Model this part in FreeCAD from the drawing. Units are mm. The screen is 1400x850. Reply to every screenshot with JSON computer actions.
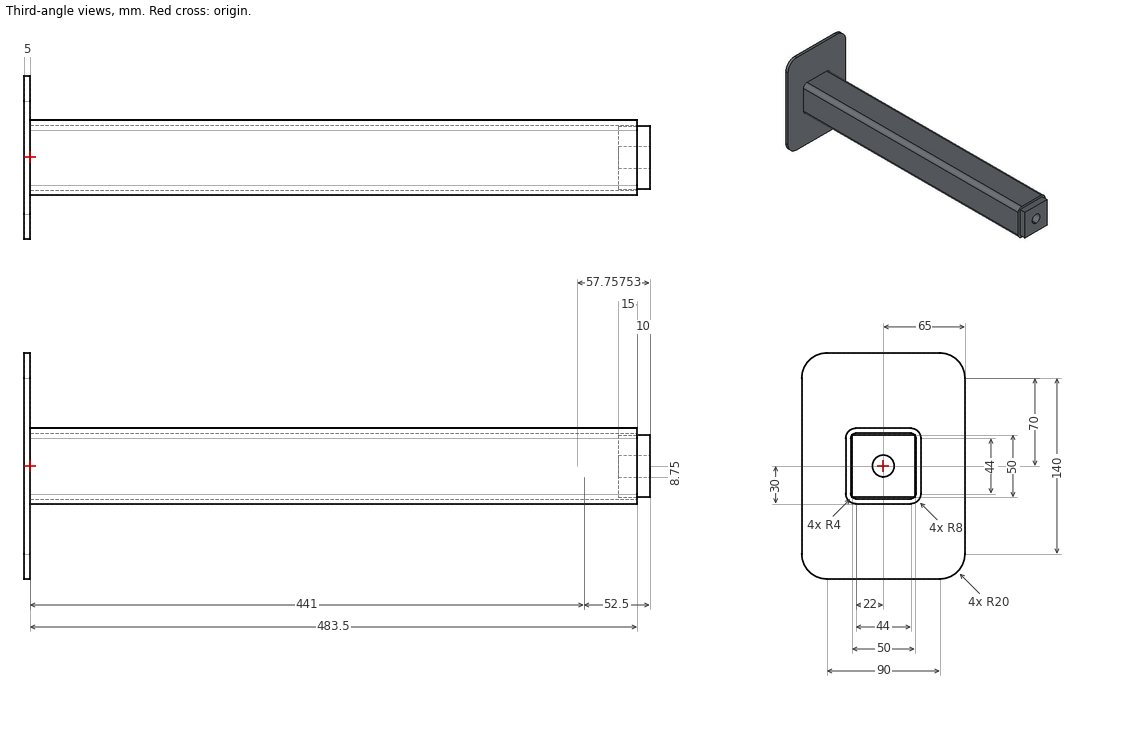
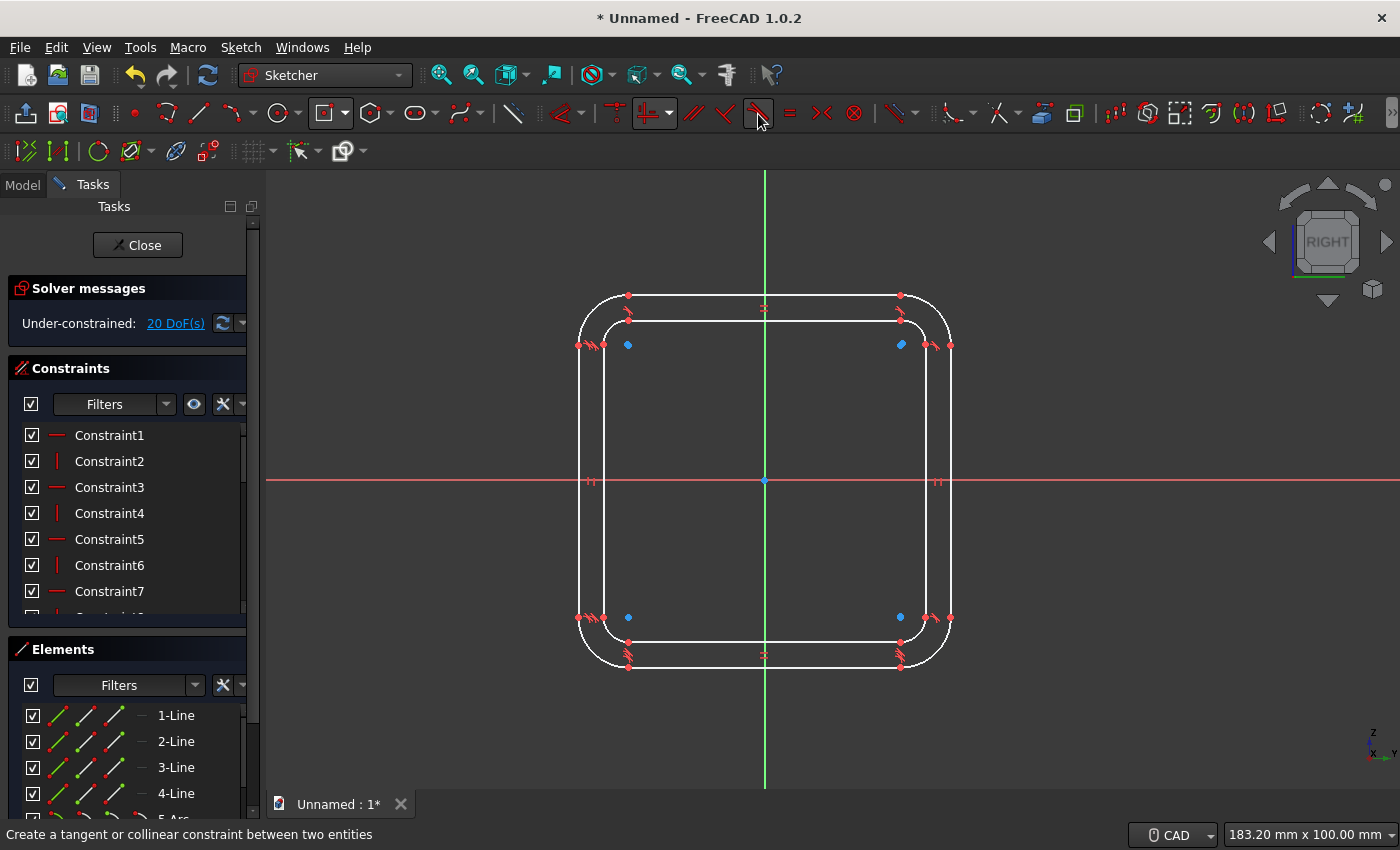
{"action": "left_click", "coordinate": [710, 321]}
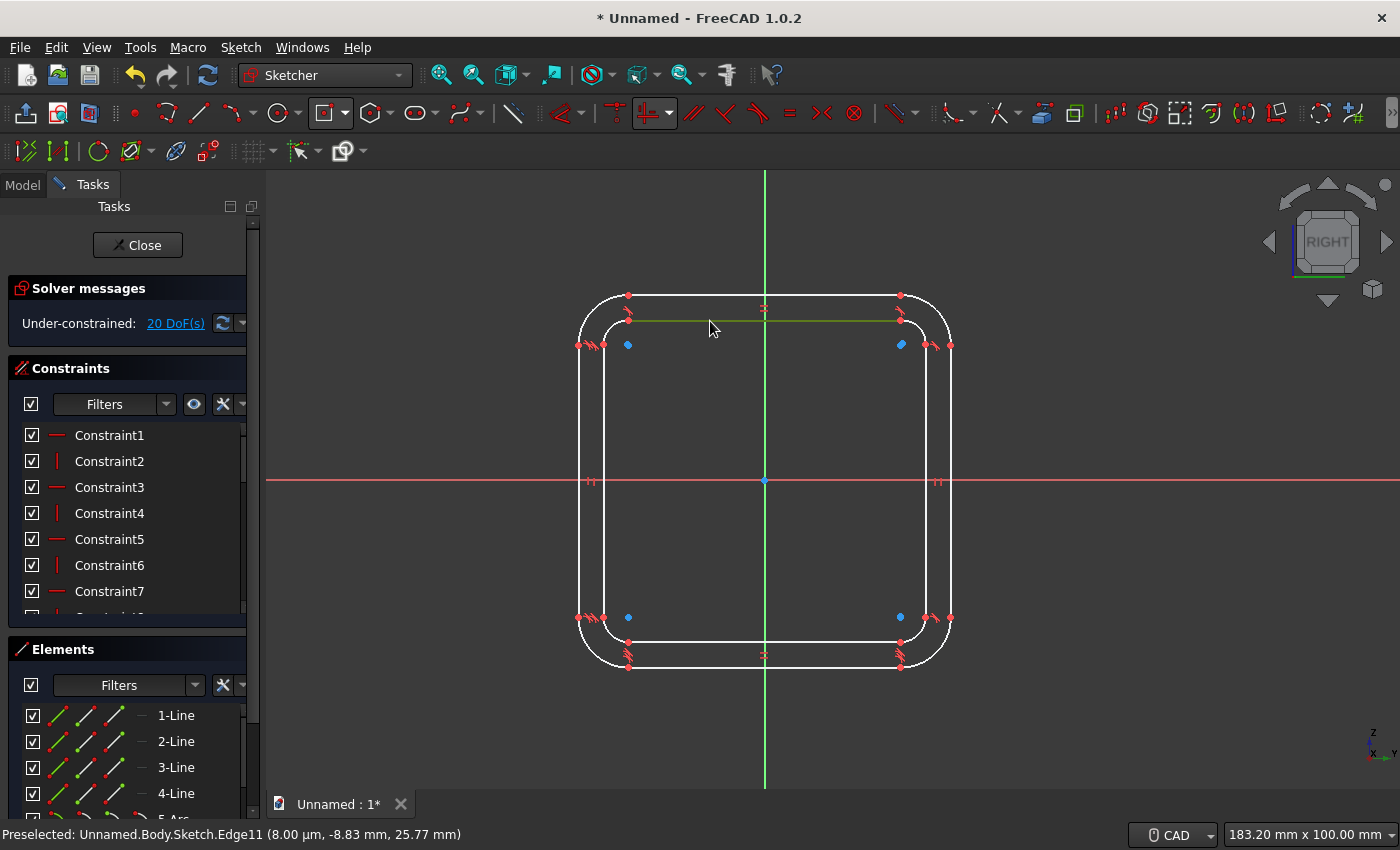
{"action": "left_click", "coordinate": [617, 323]}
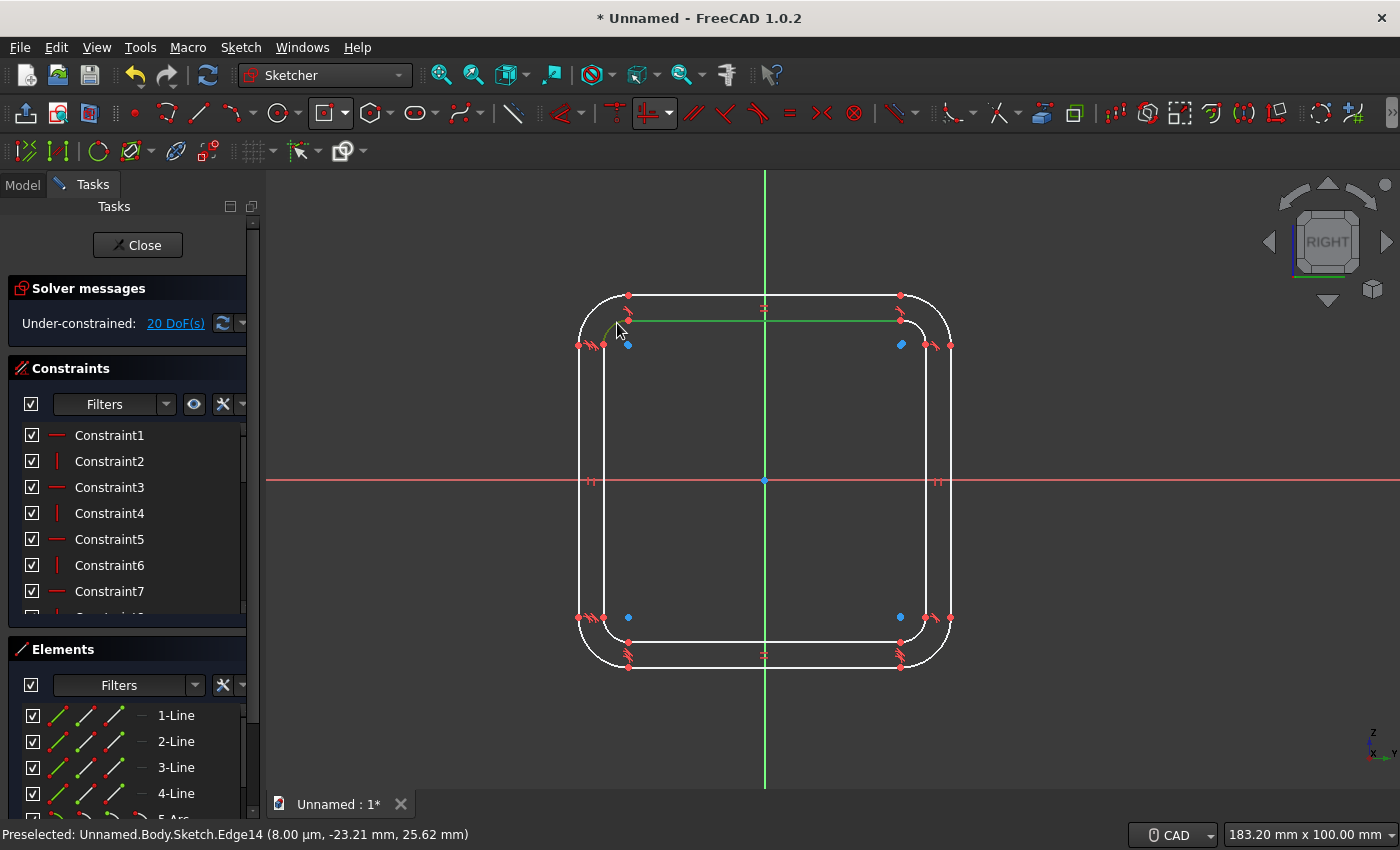
{"action": "left_click", "coordinate": [758, 114]}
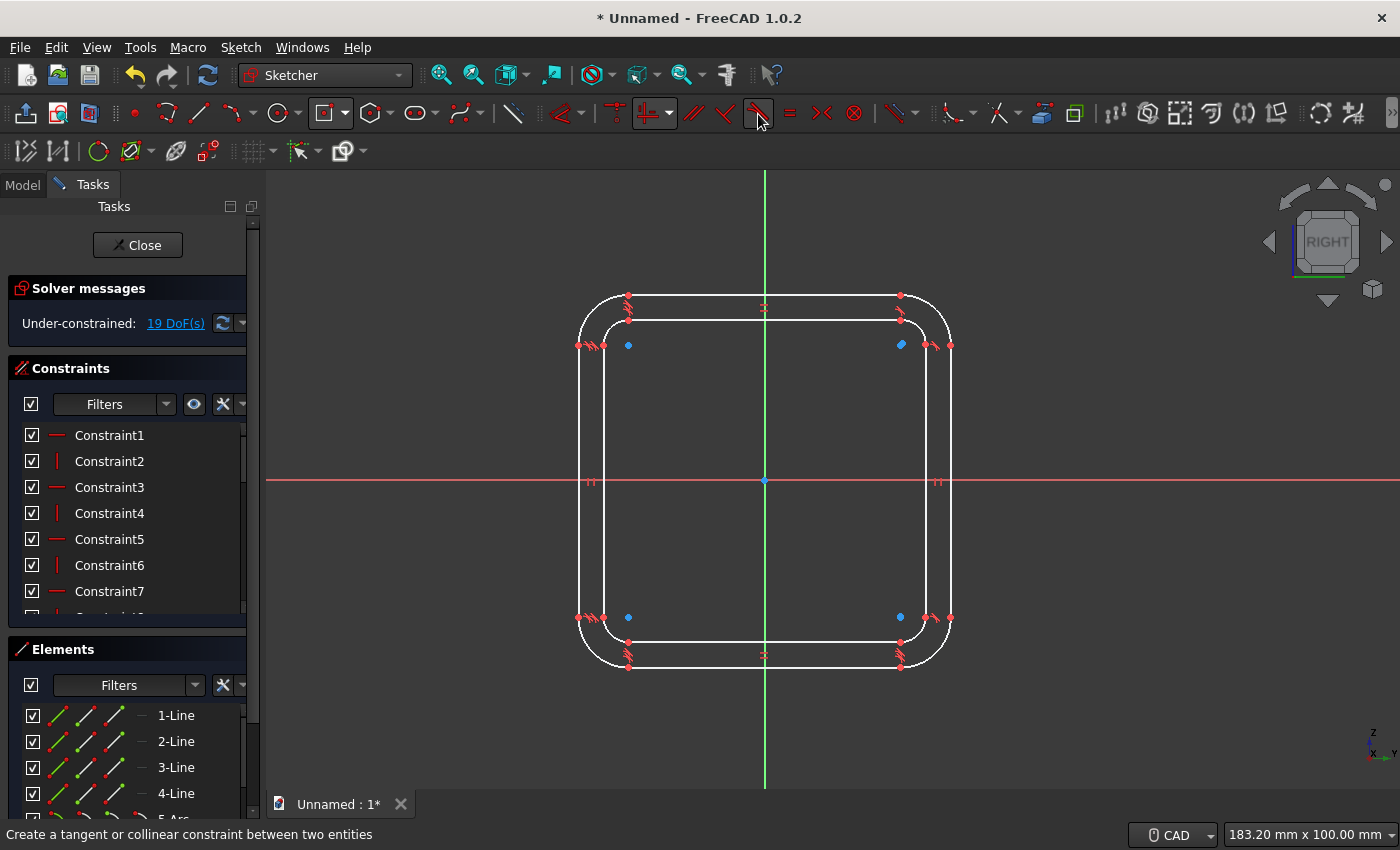
{"action": "left_click", "coordinate": [710, 320]}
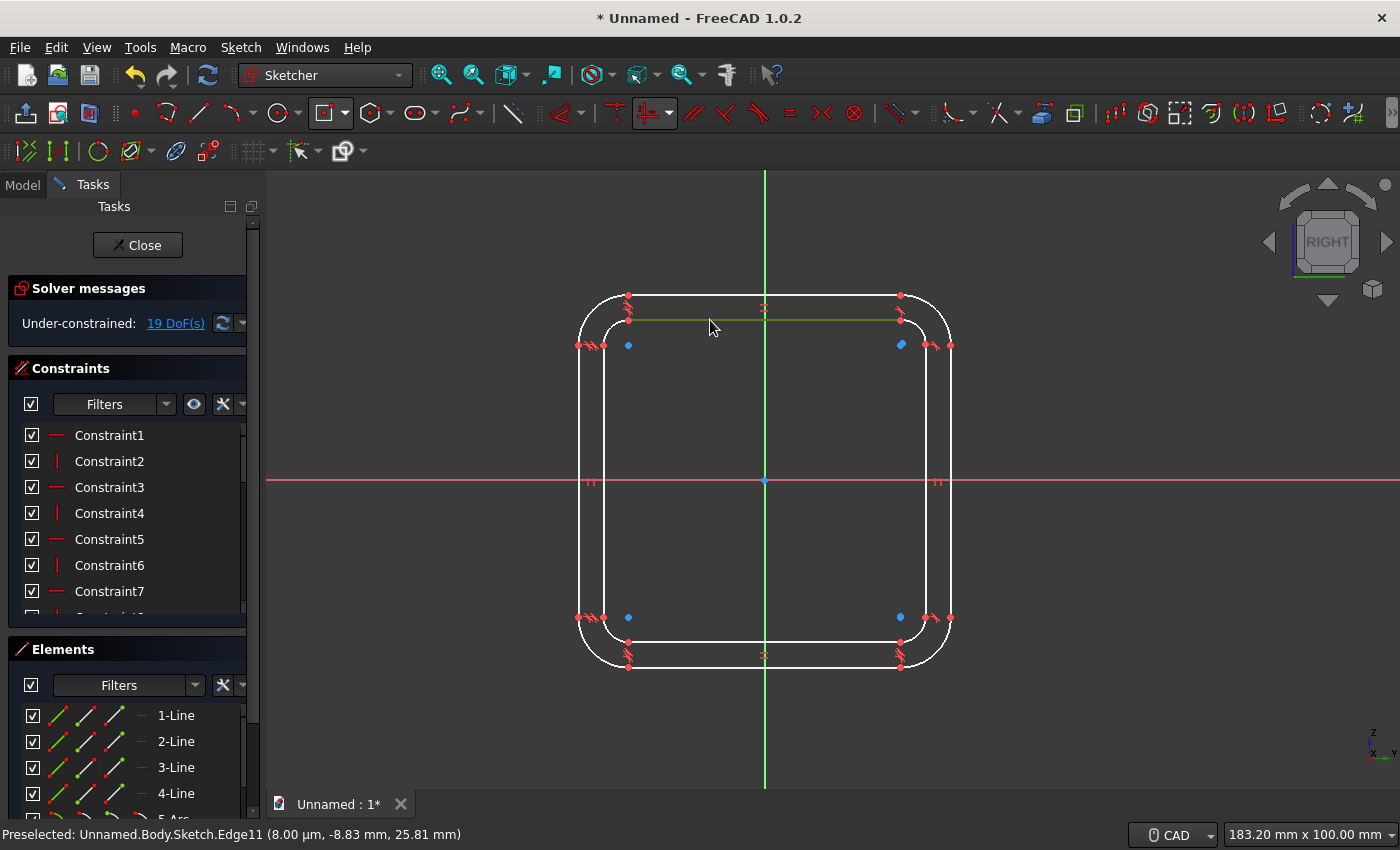
{"action": "left_click", "coordinate": [923, 333]}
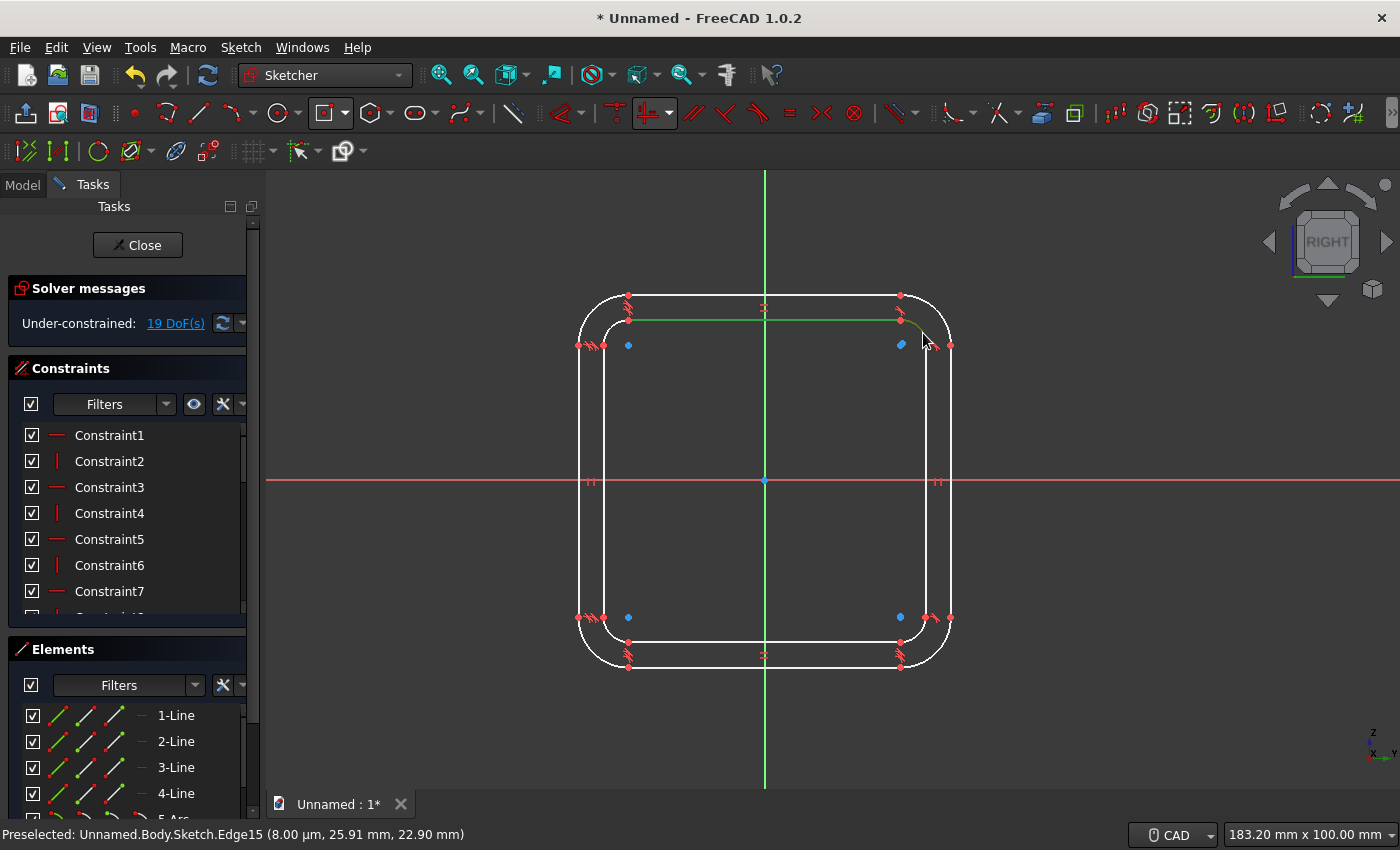
{"action": "left_click", "coordinate": [758, 114]}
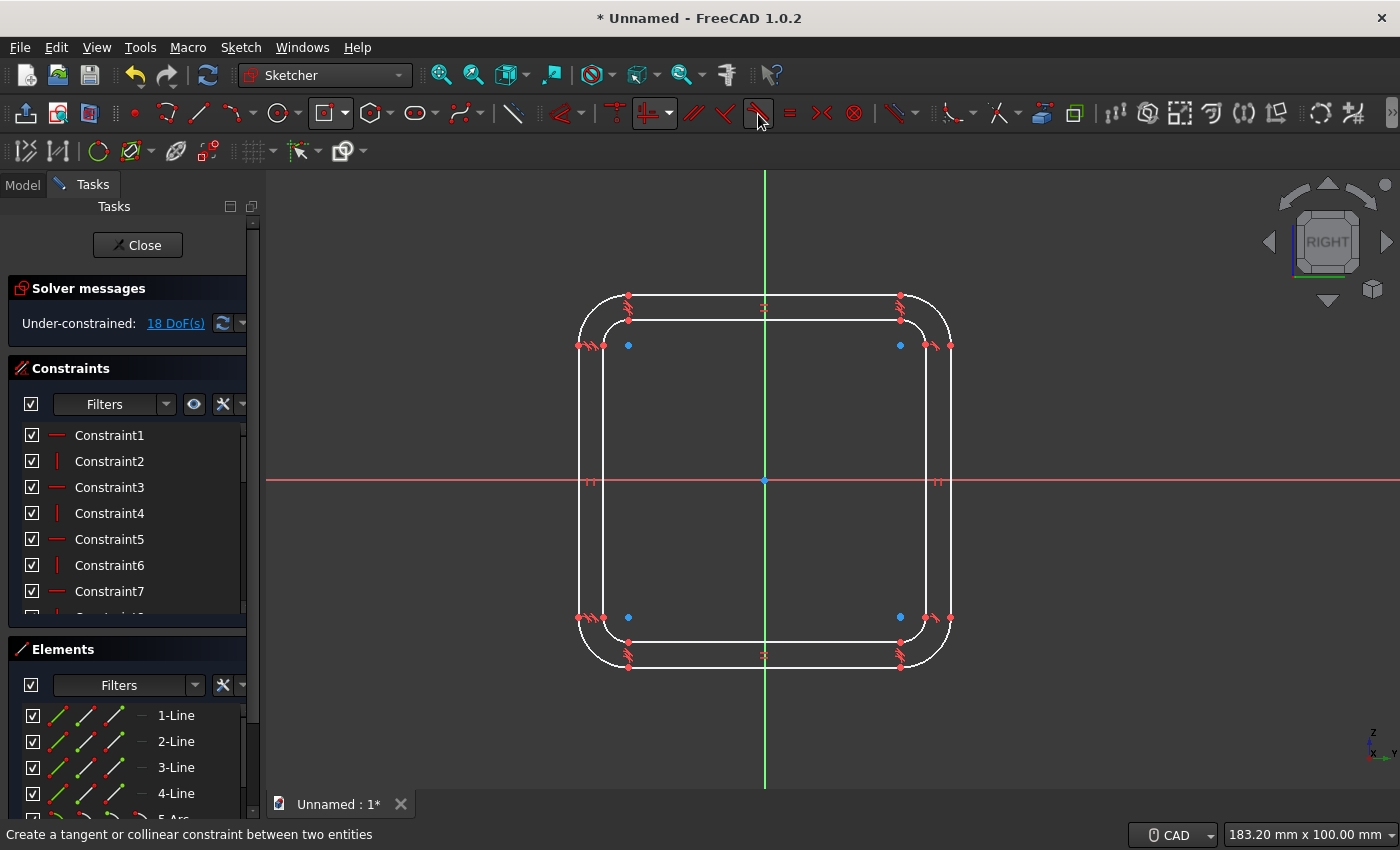
{"action": "left_click", "coordinate": [926, 426]}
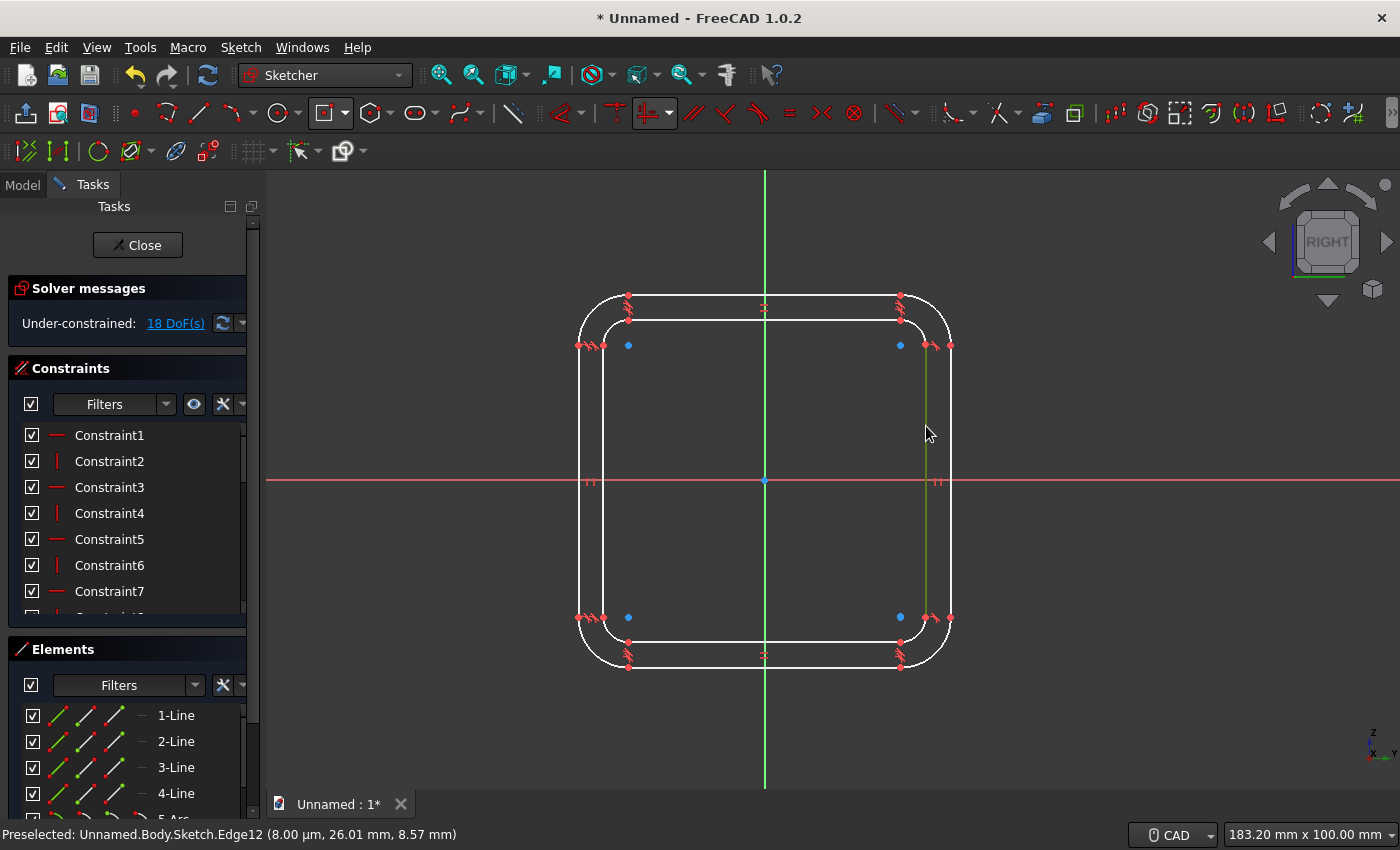
{"action": "left_click", "coordinate": [923, 333]}